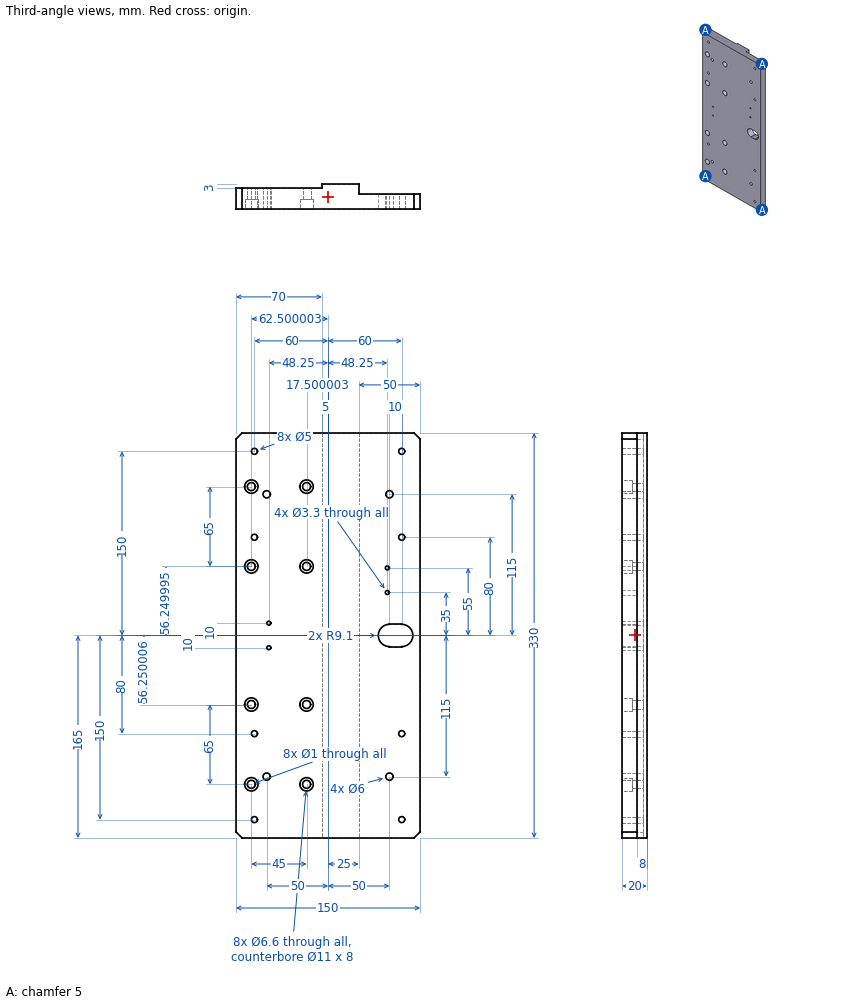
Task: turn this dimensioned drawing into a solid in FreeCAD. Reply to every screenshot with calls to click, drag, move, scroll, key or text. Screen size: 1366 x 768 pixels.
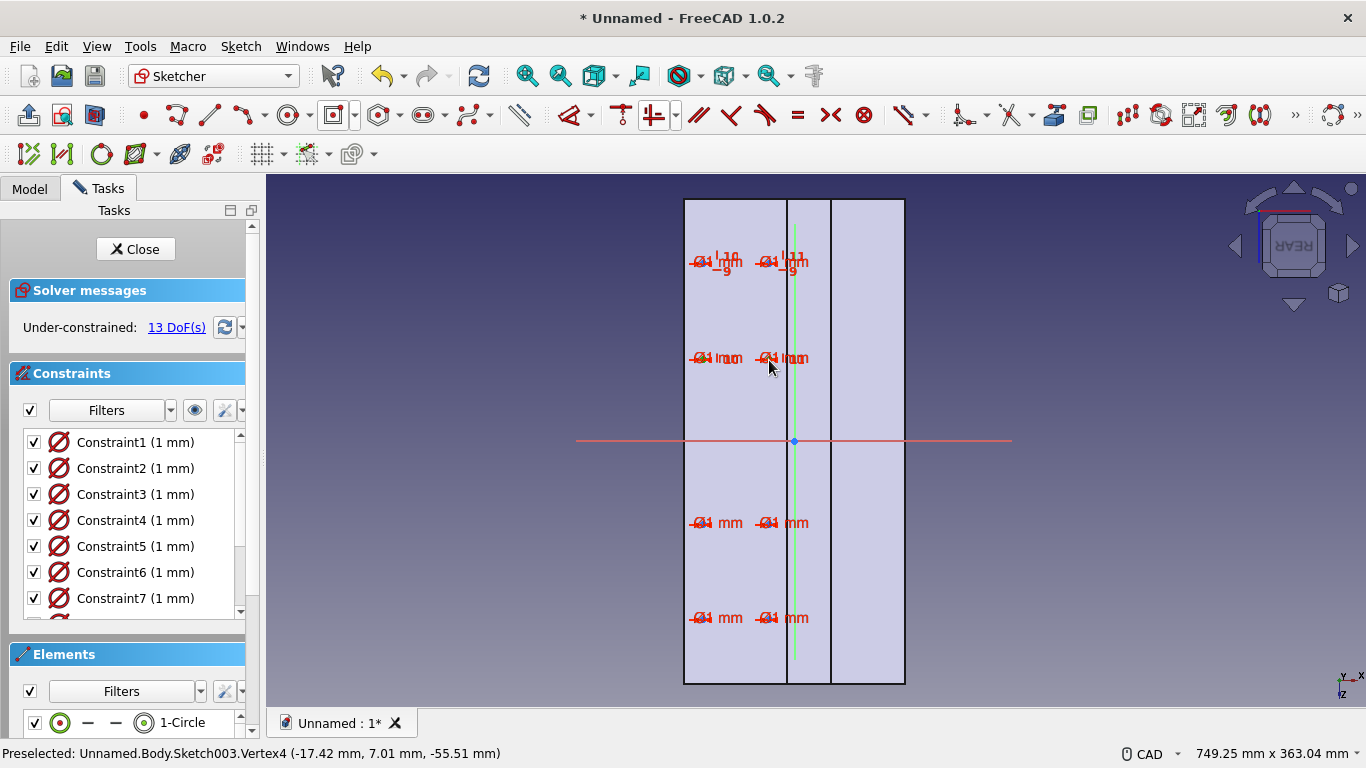
key(h)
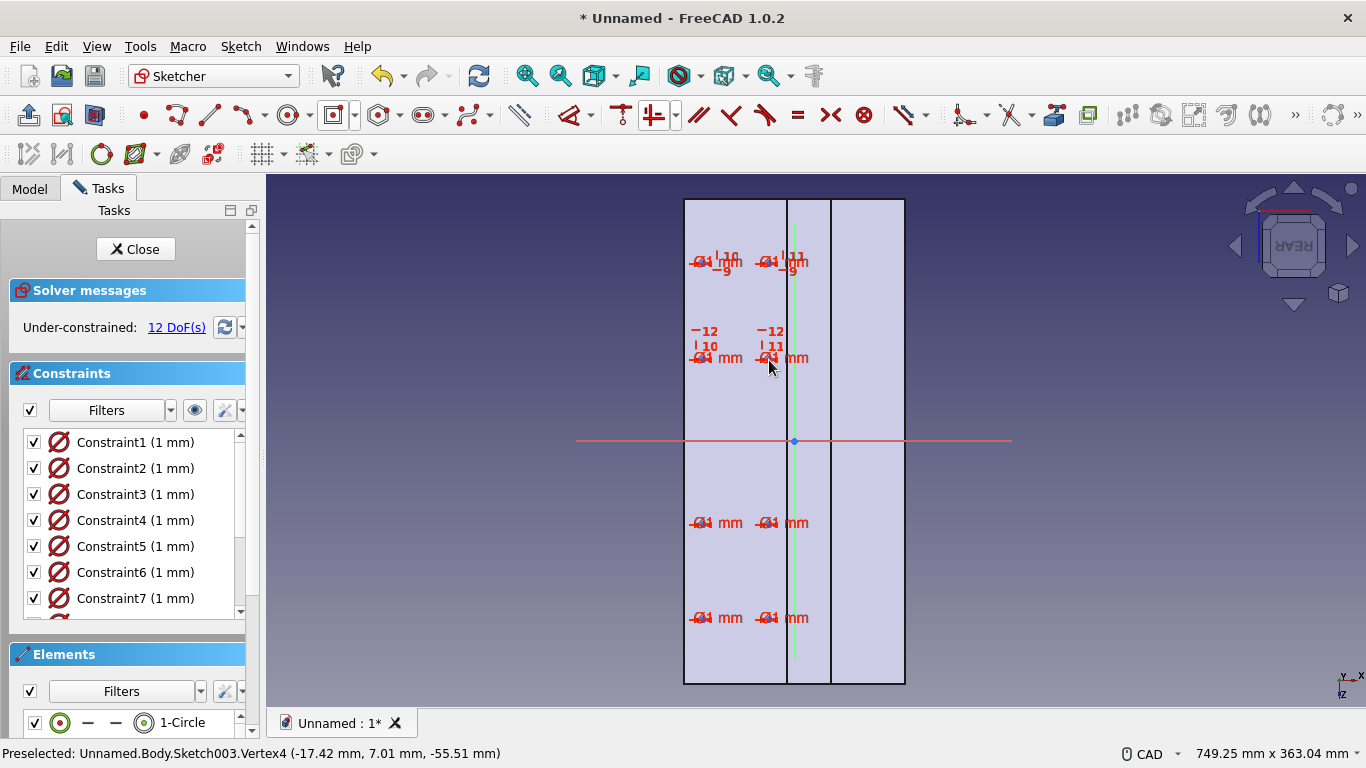
click(703, 525)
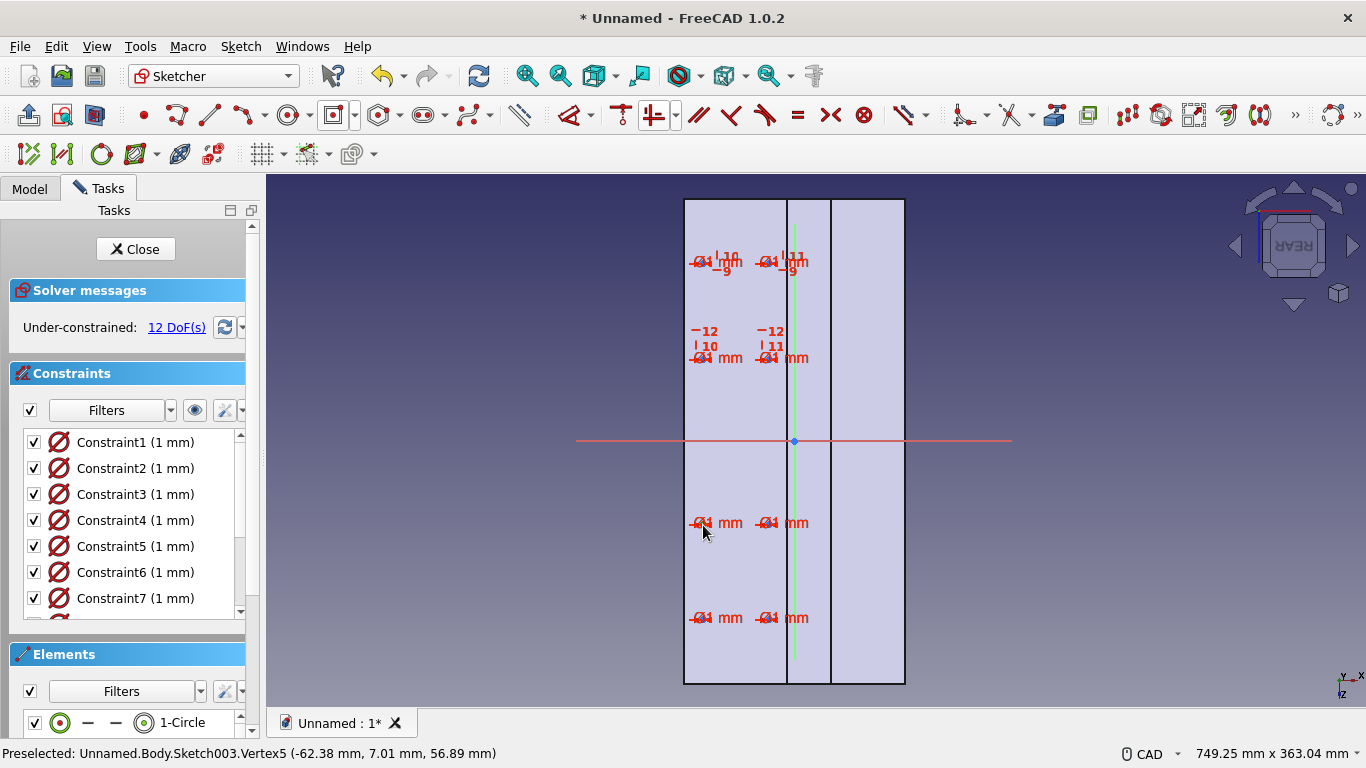
click(769, 525)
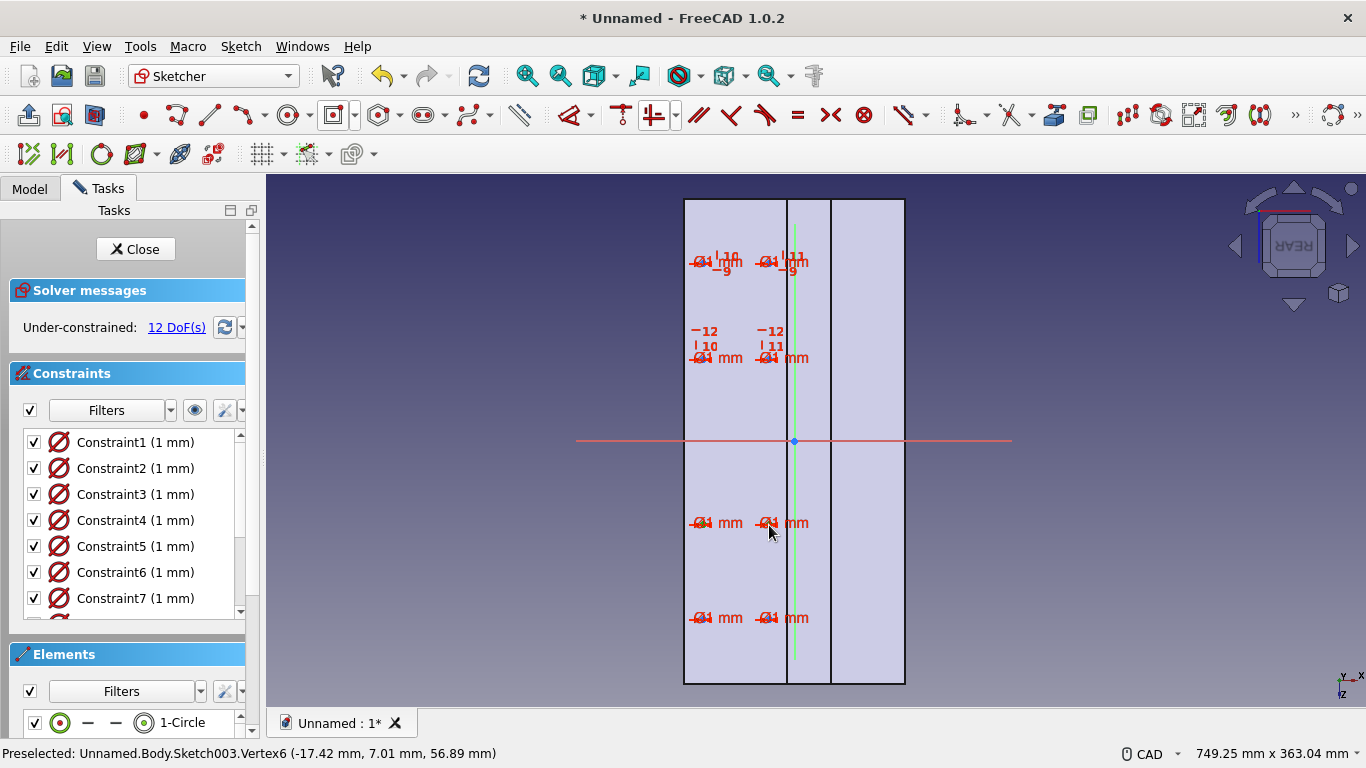
click(676, 116)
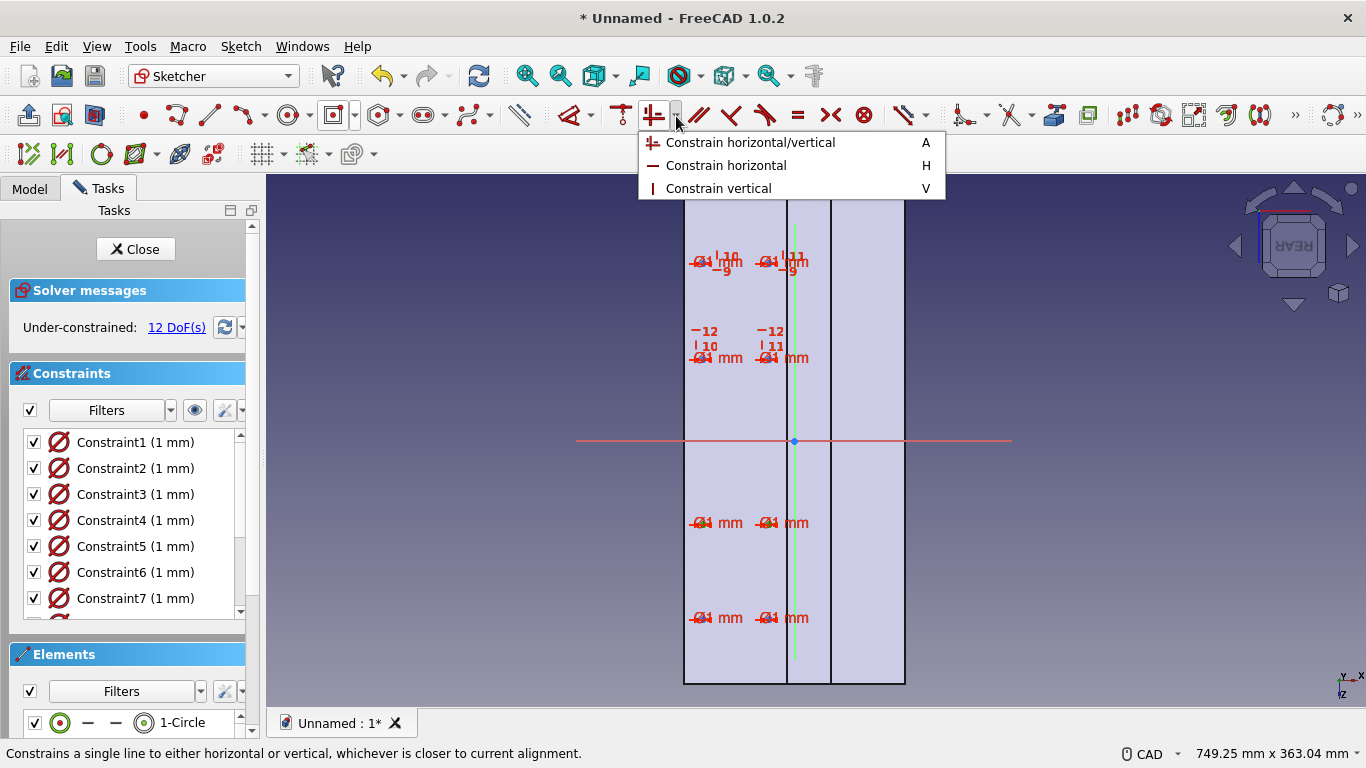
click(792, 166)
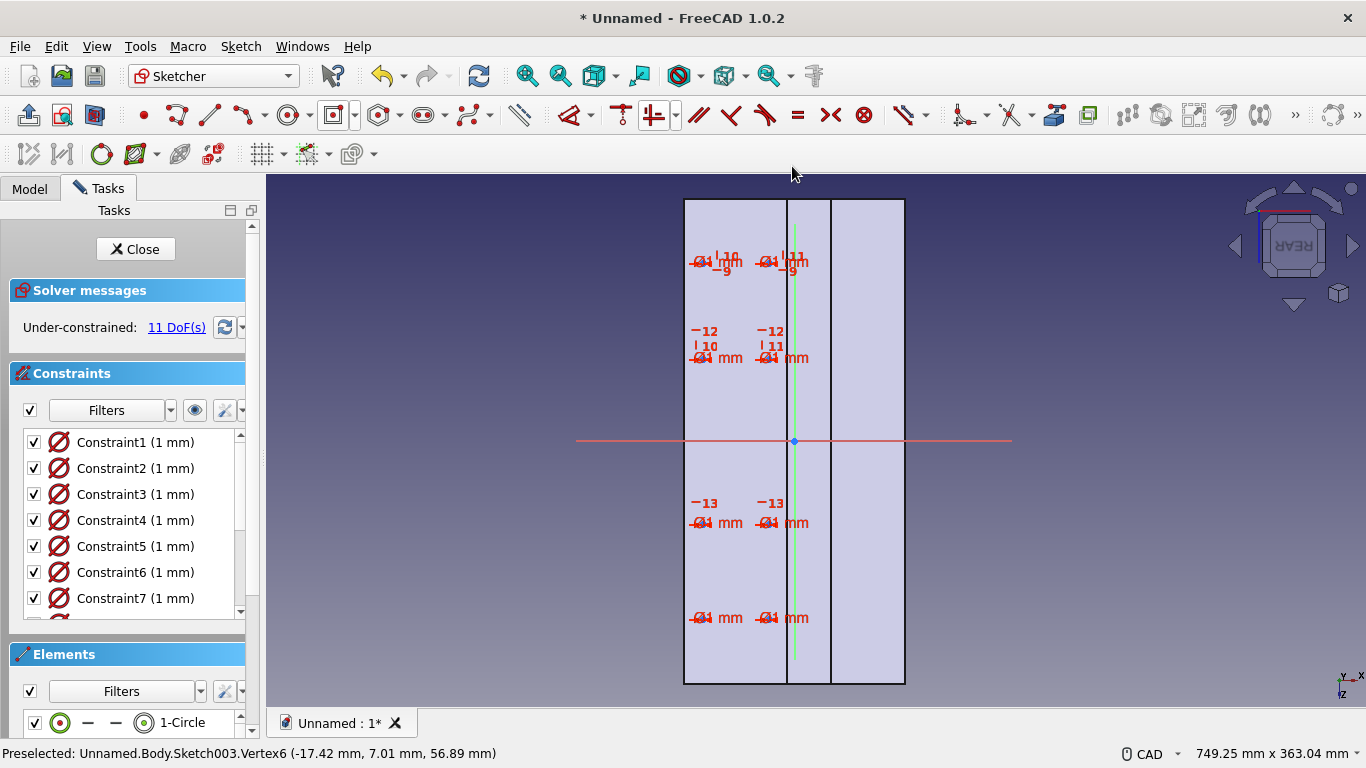
click(703, 525)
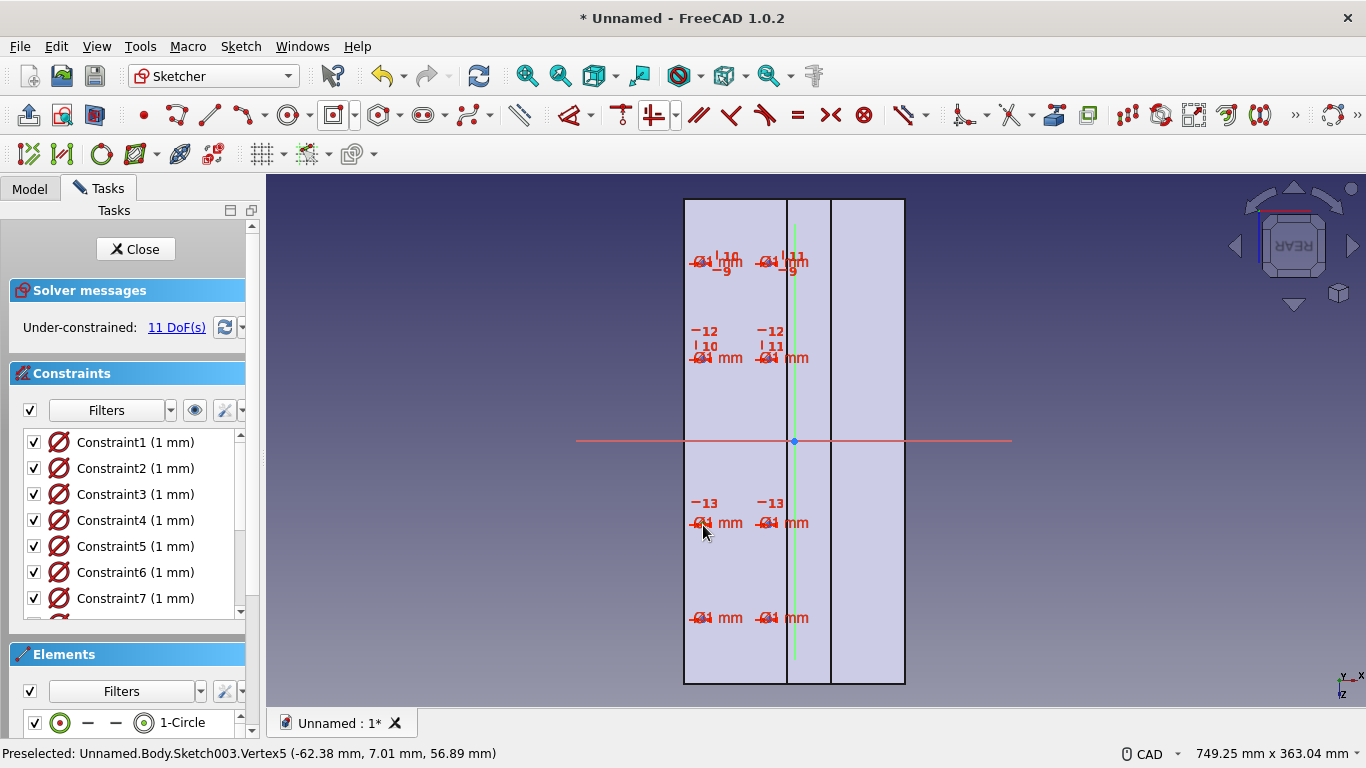
click(703, 620)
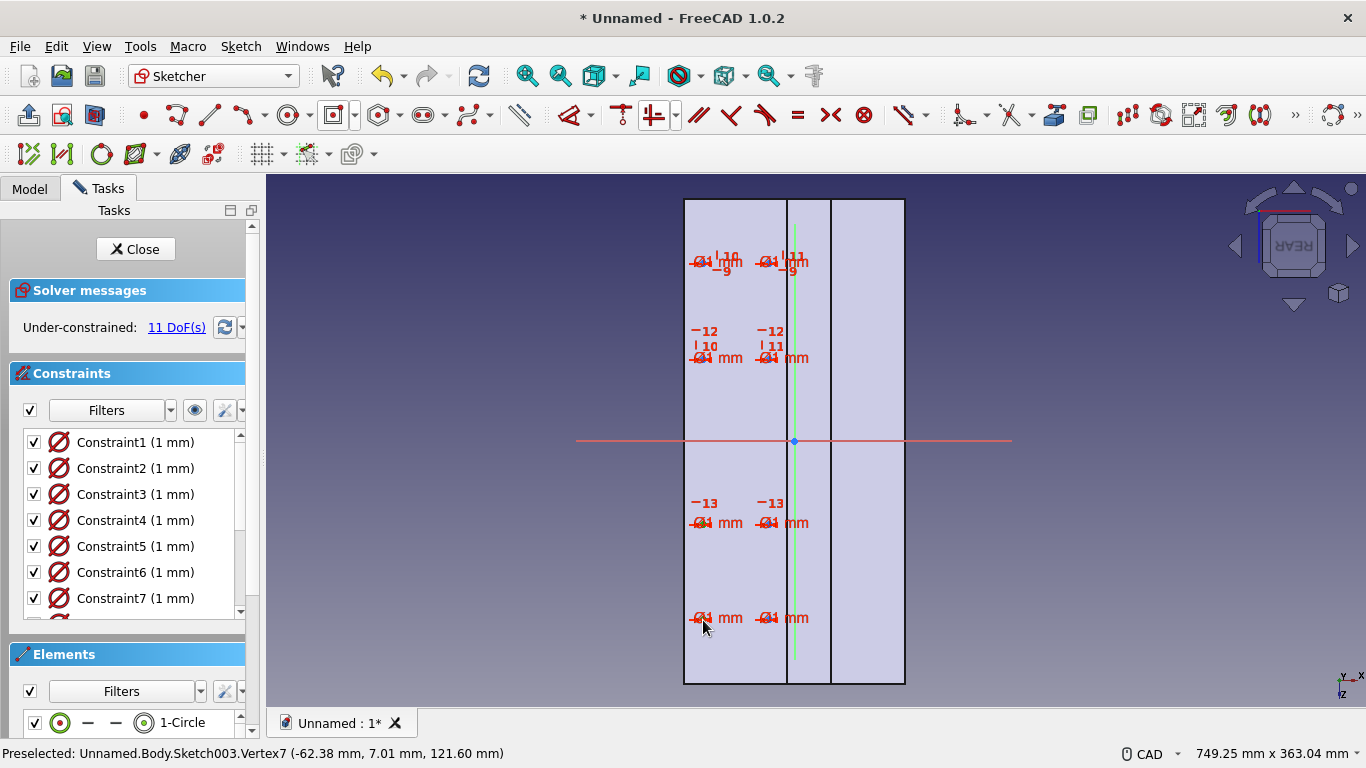
click(676, 116)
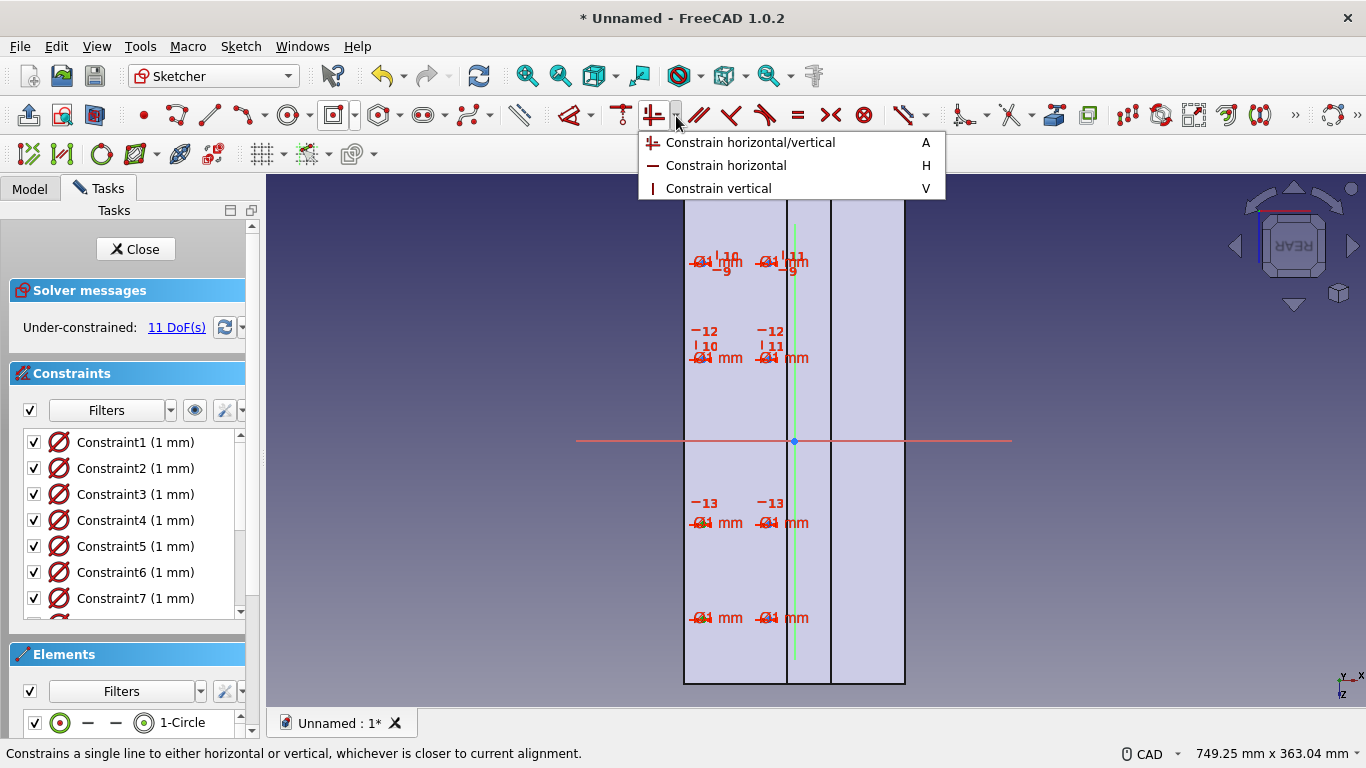
click(792, 188)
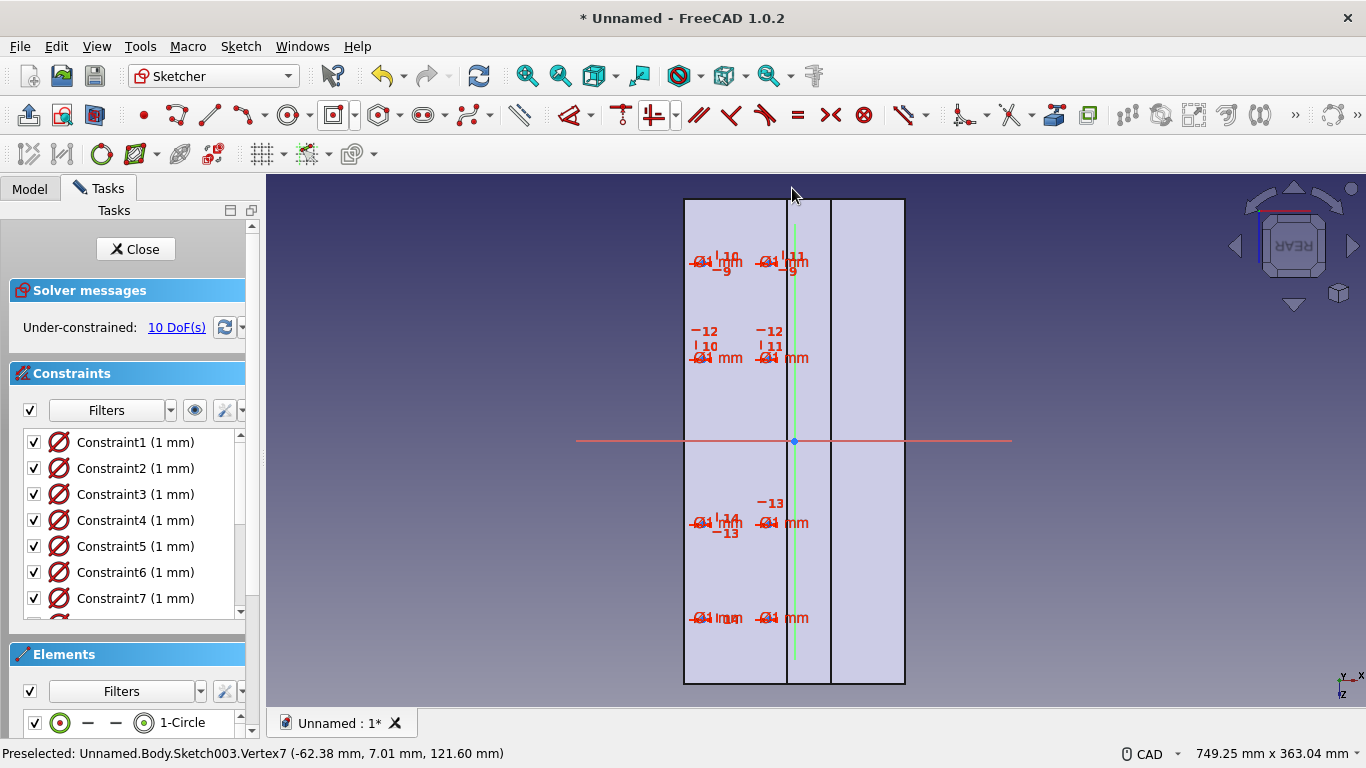
click(769, 525)